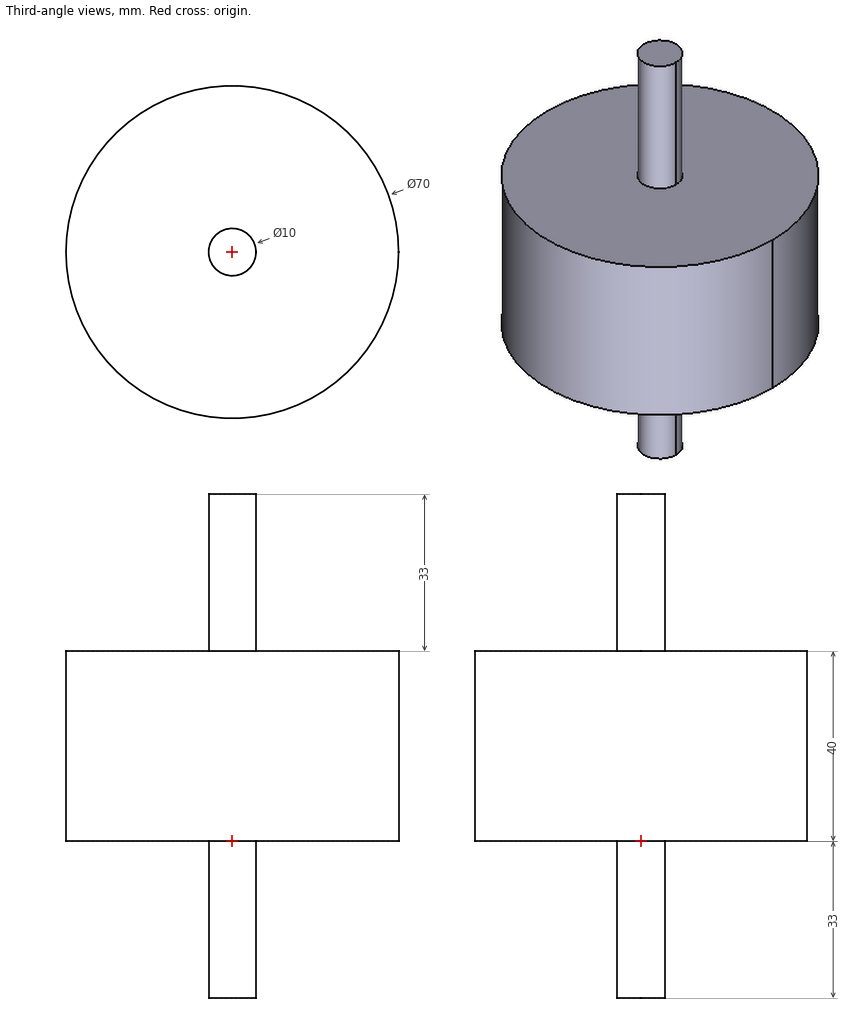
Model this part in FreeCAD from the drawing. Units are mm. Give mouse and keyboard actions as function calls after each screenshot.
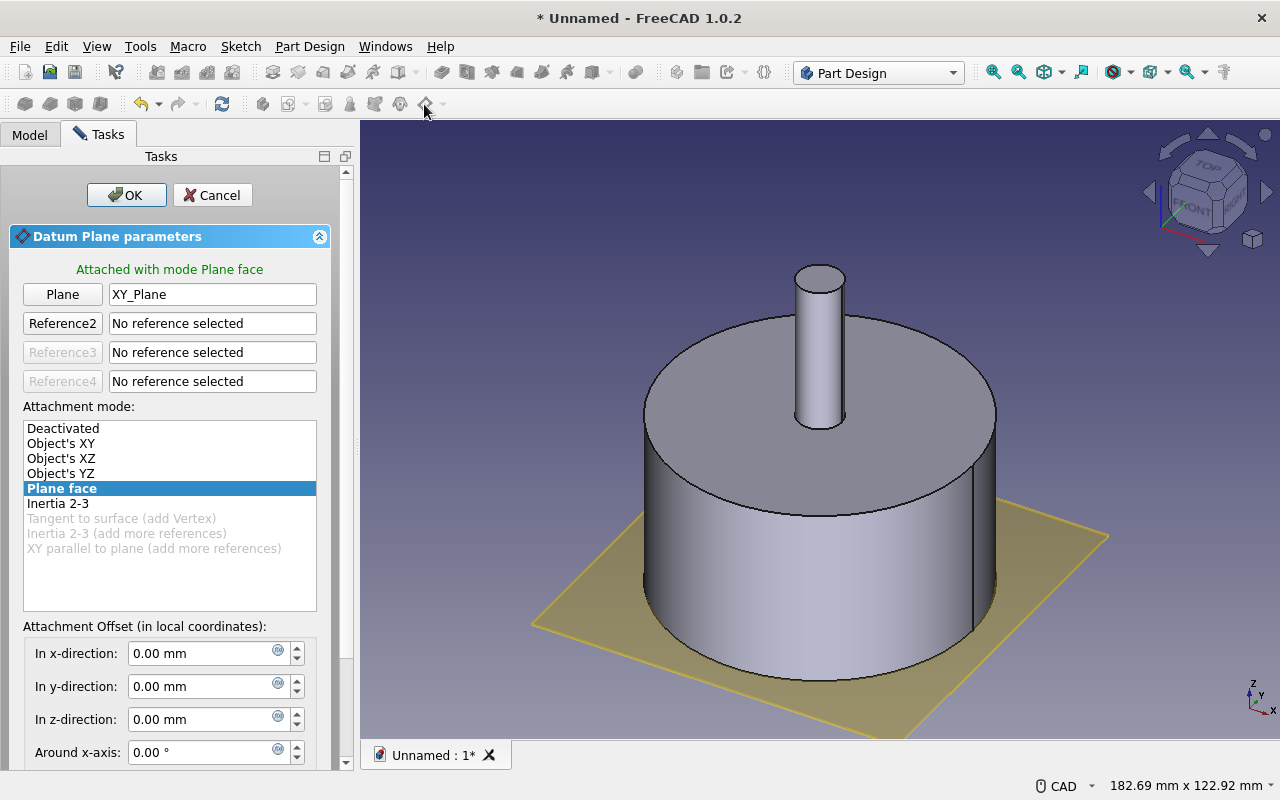
triple_click(210, 720)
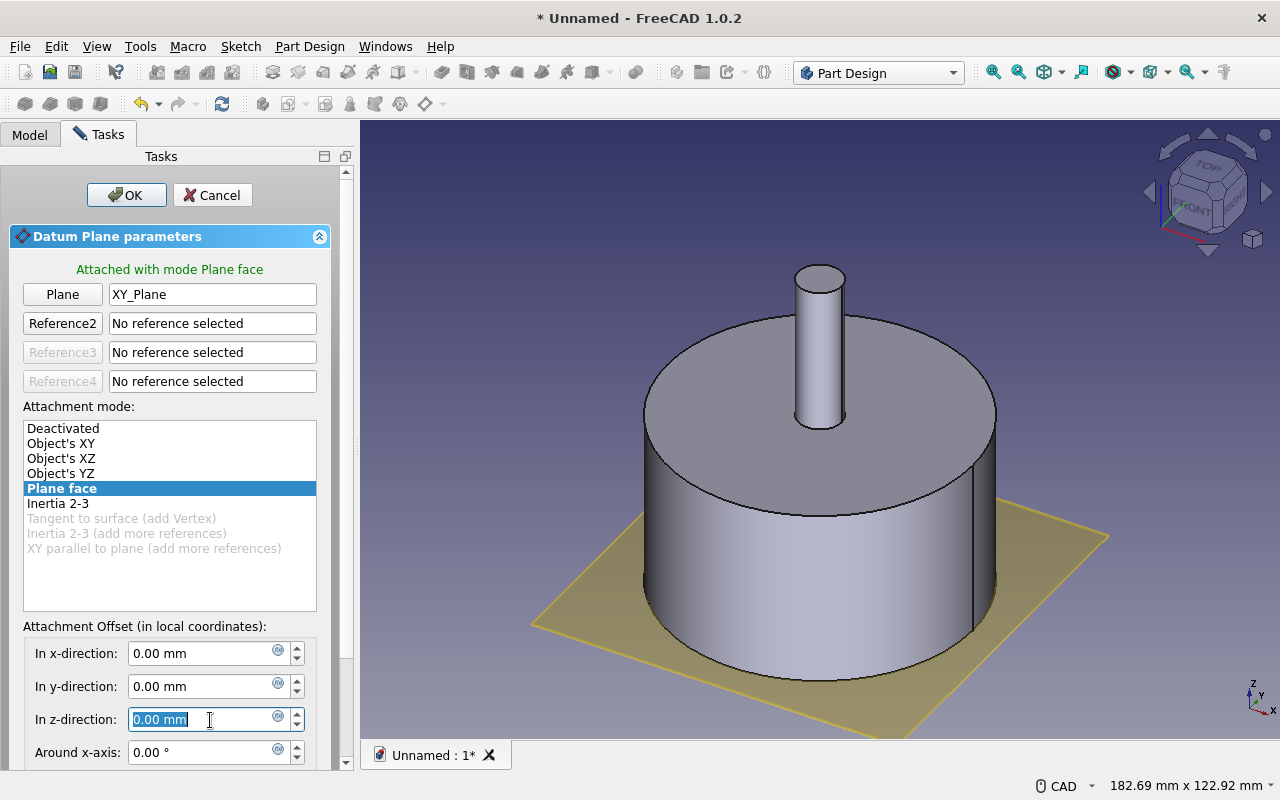
text(-33)
key(Tab)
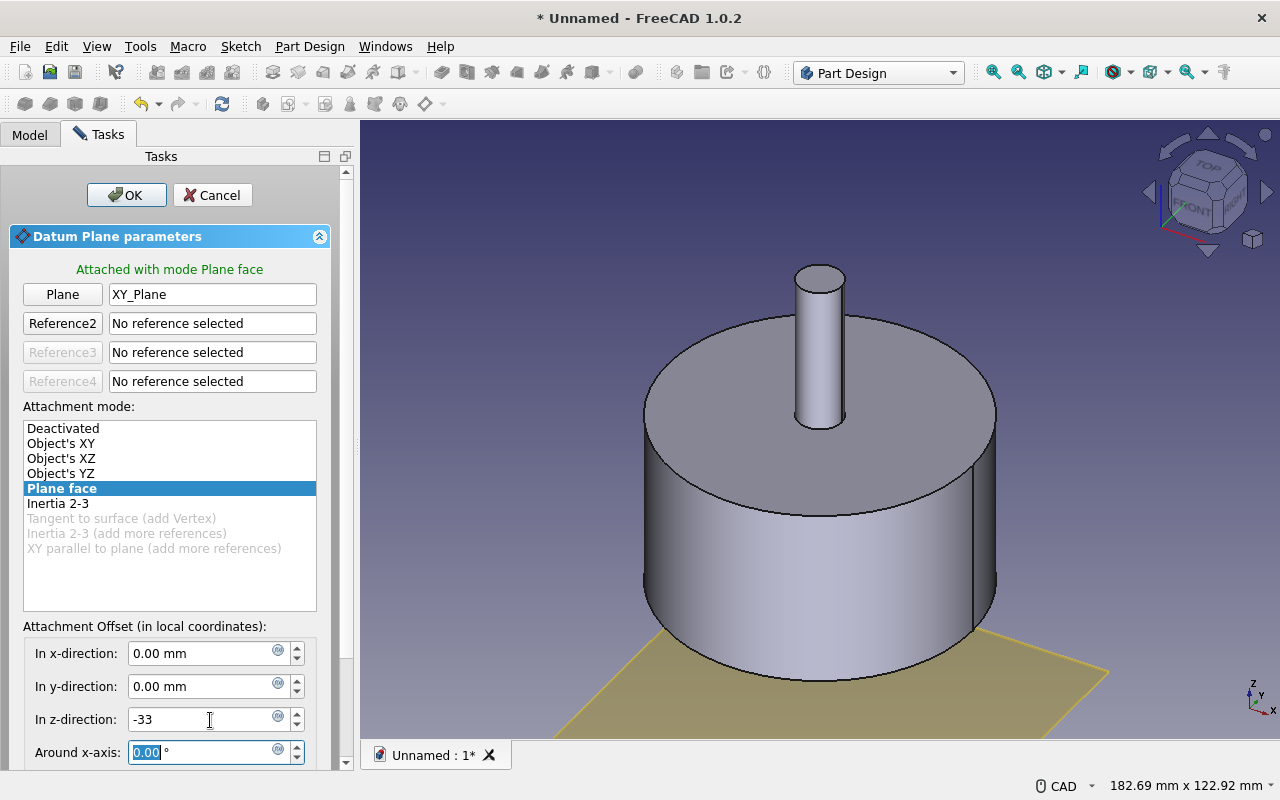
click(127, 195)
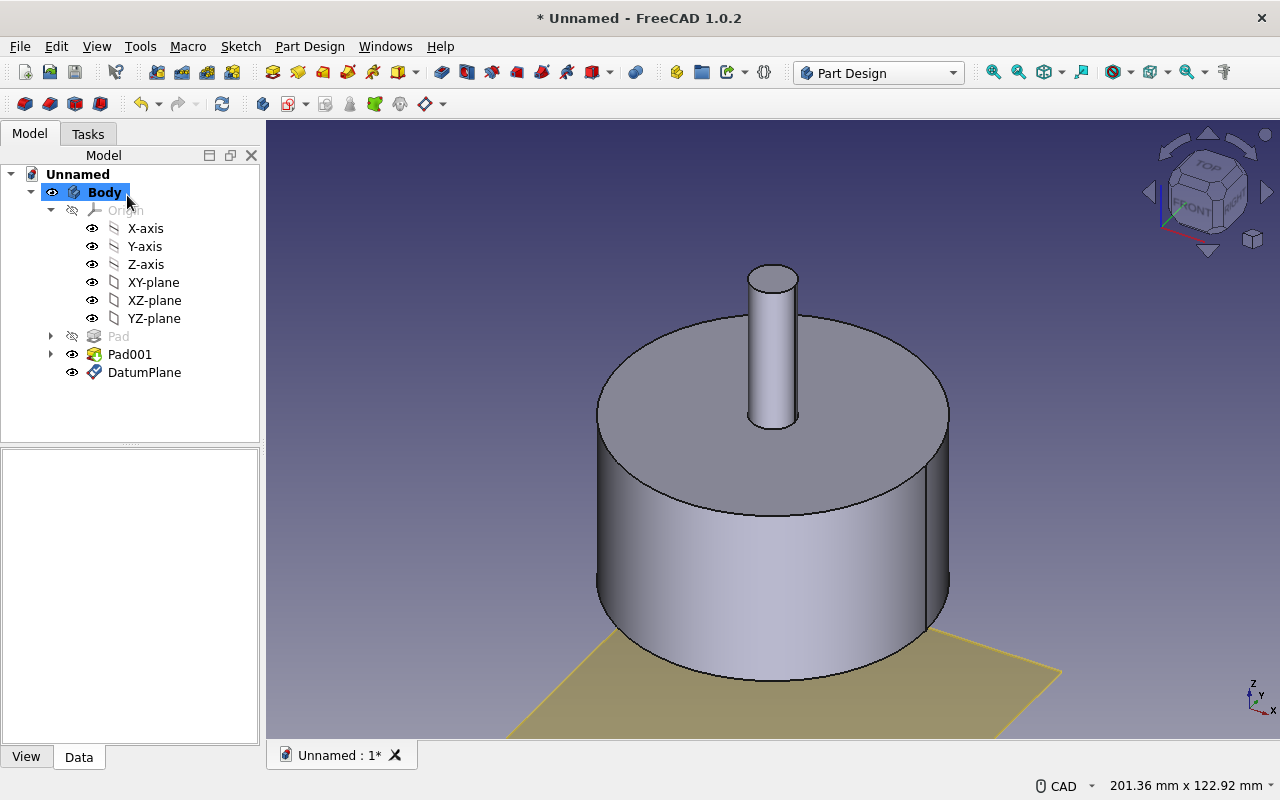
click(117, 372)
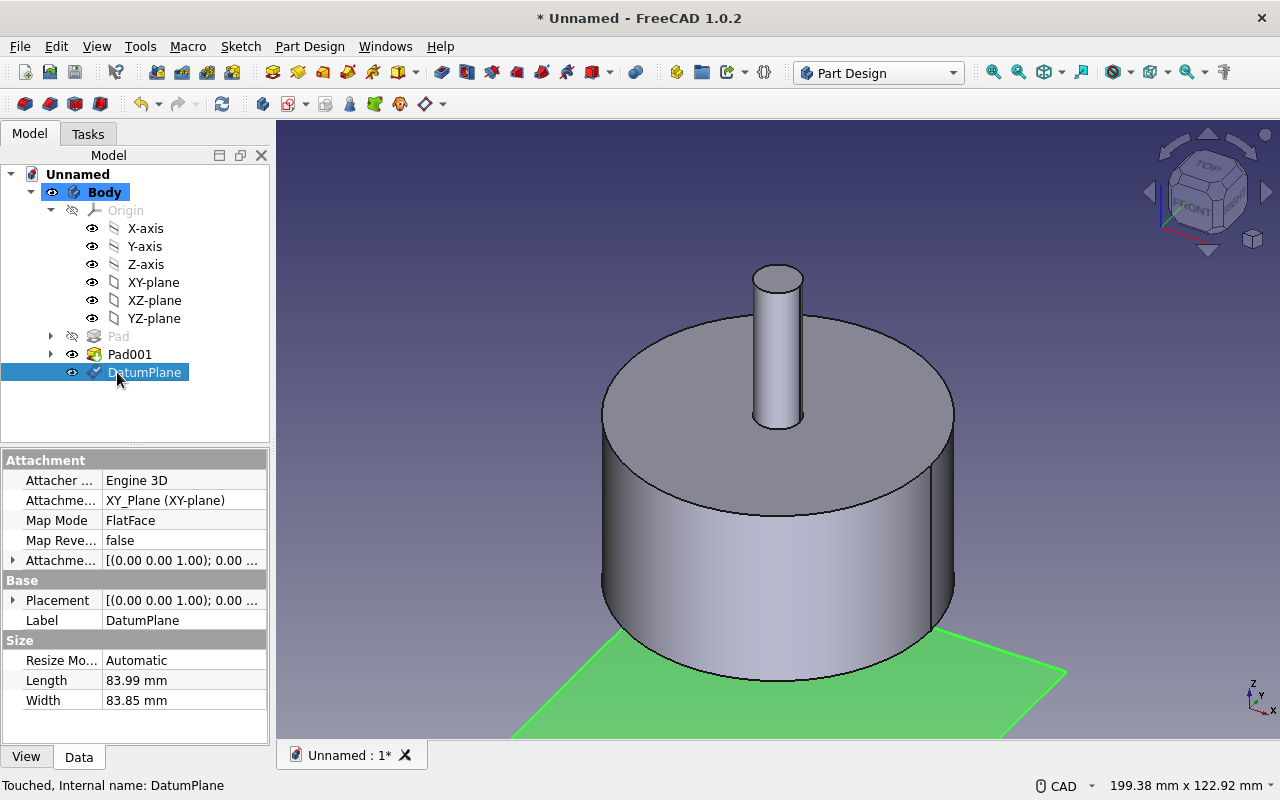
click(288, 104)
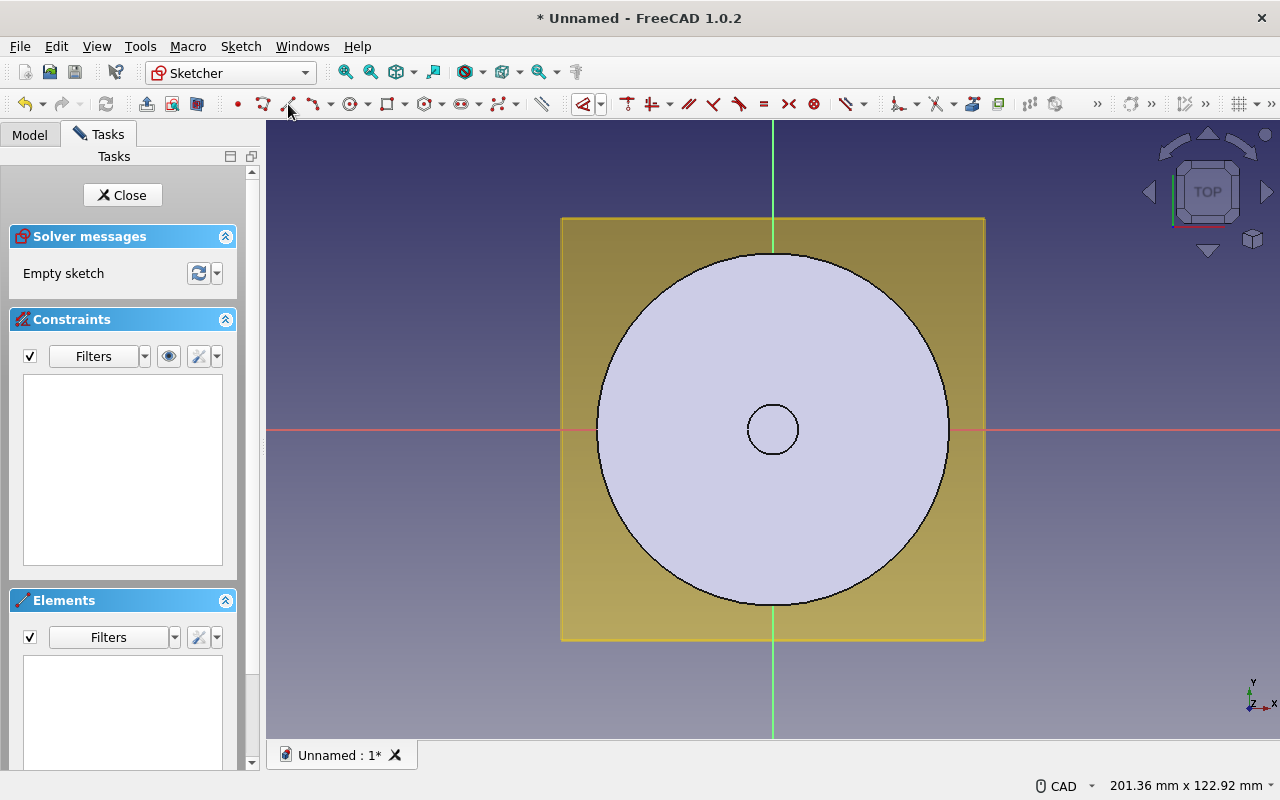
key(q)
key(s)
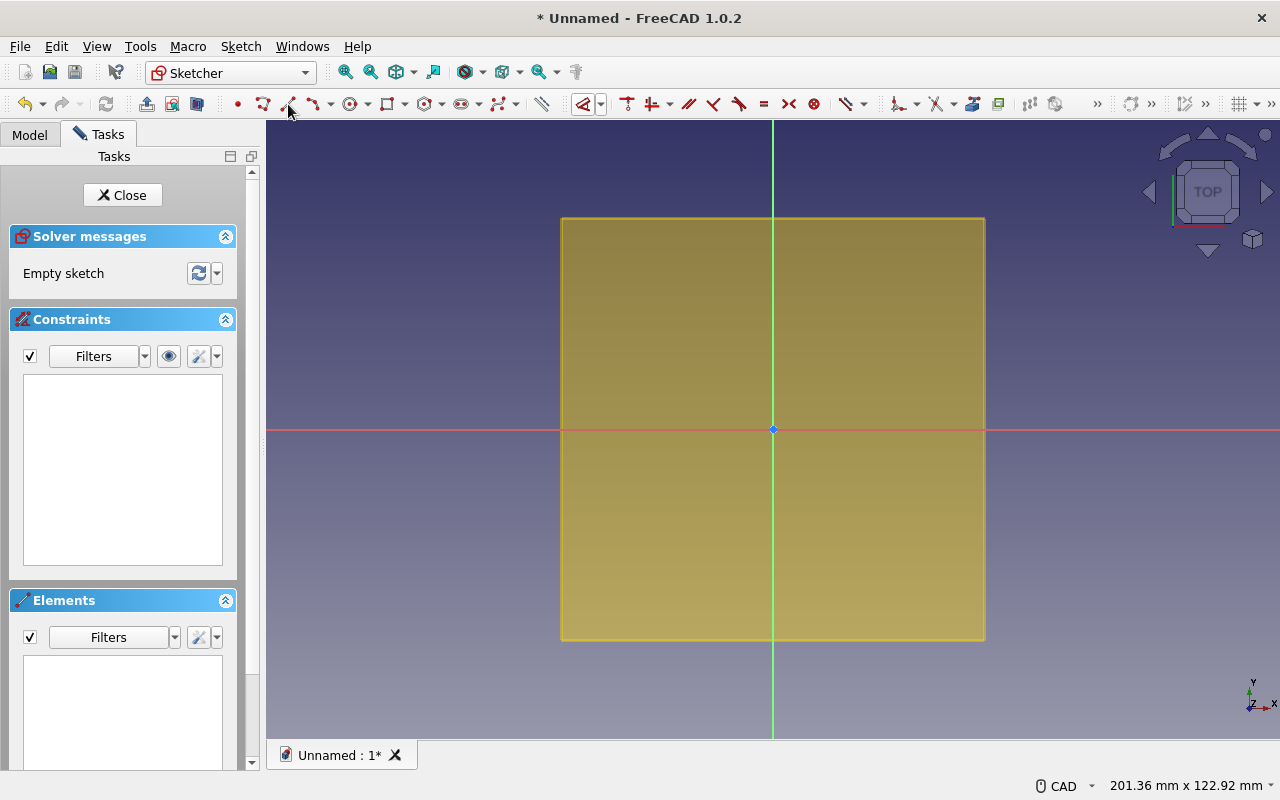
scroll(784, 430, up, 10)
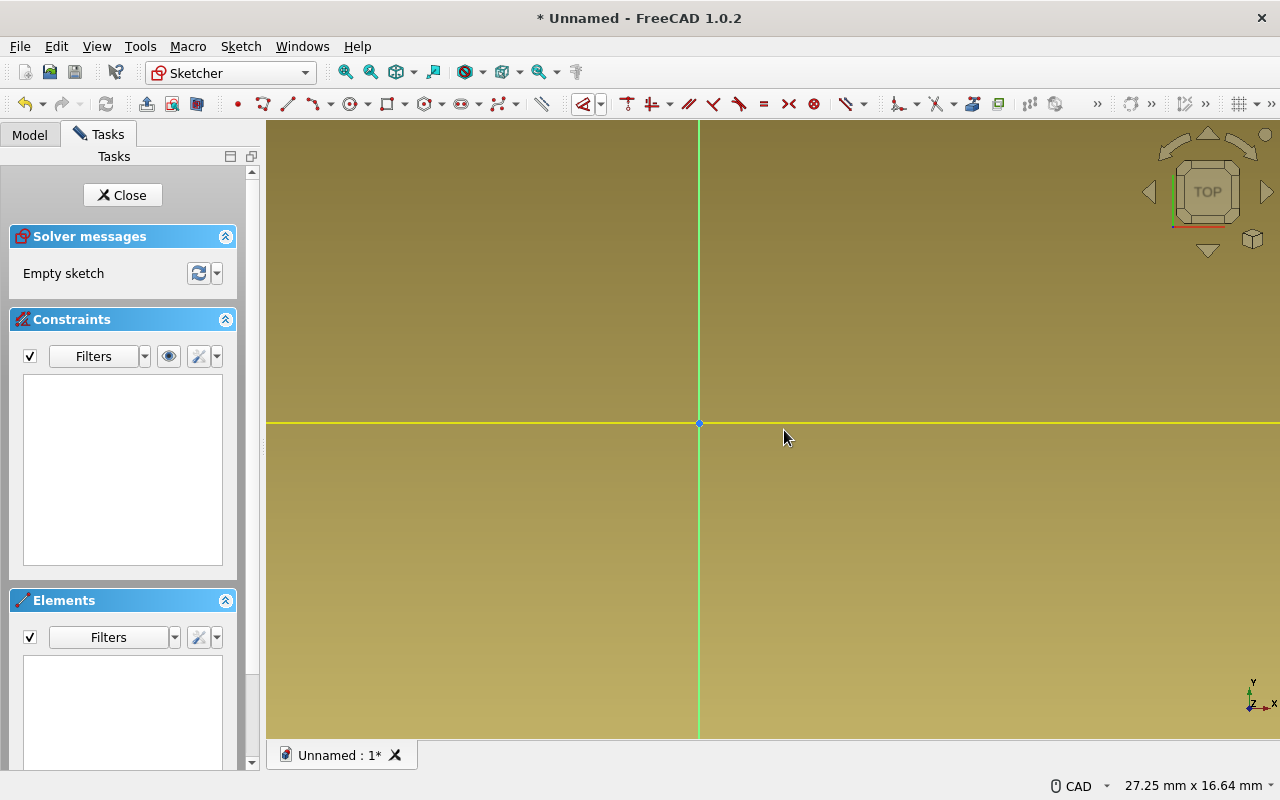
click(350, 104)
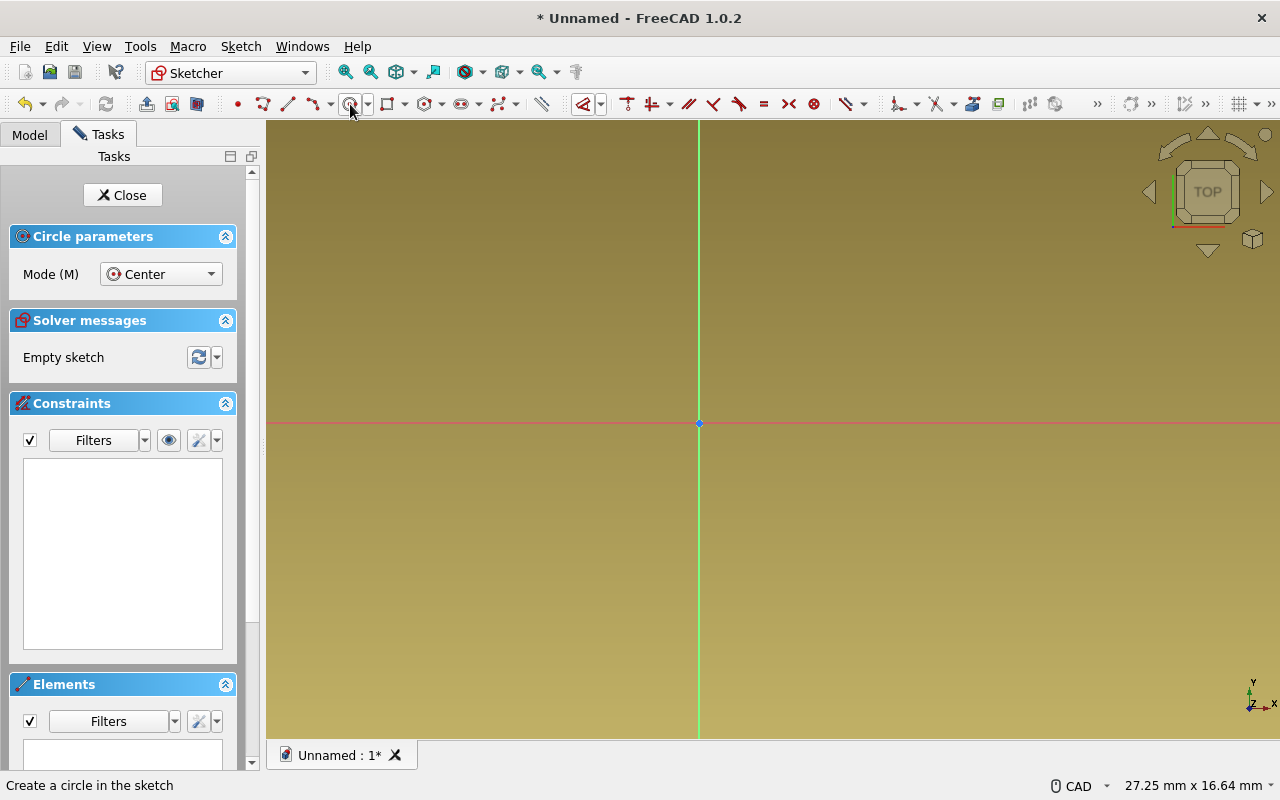
click(699, 423)
click(831, 292)
key(Escape)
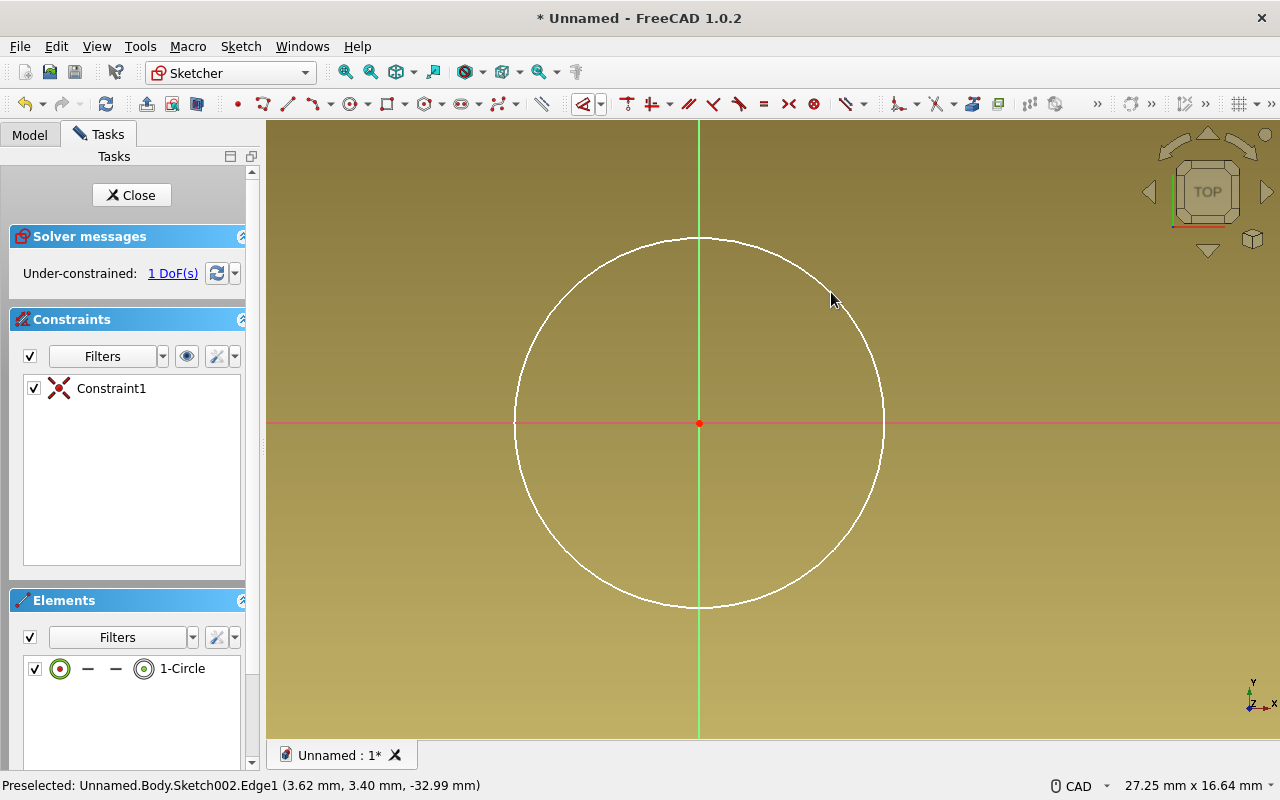
key(d)